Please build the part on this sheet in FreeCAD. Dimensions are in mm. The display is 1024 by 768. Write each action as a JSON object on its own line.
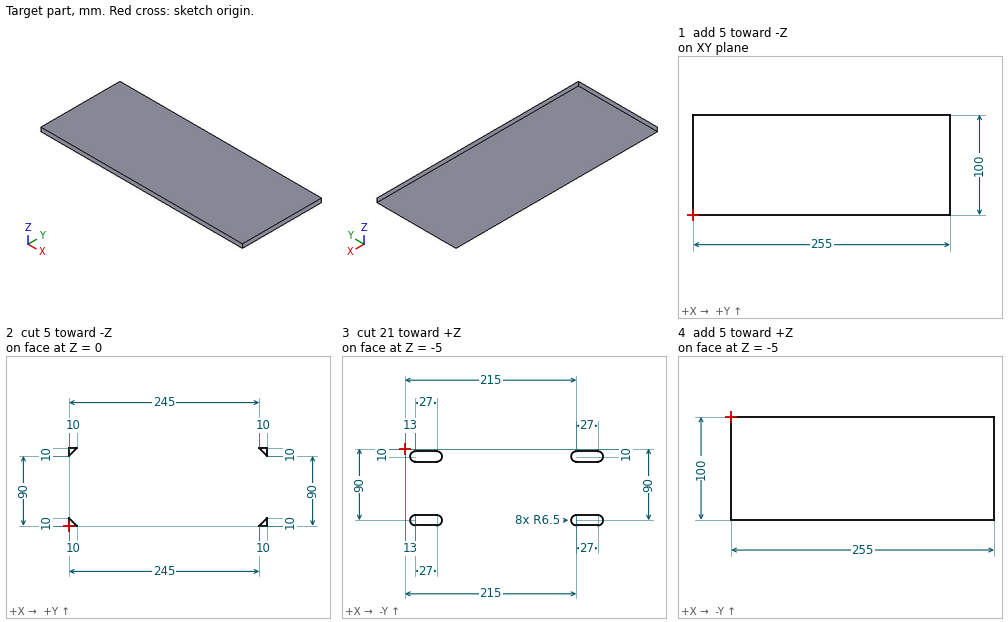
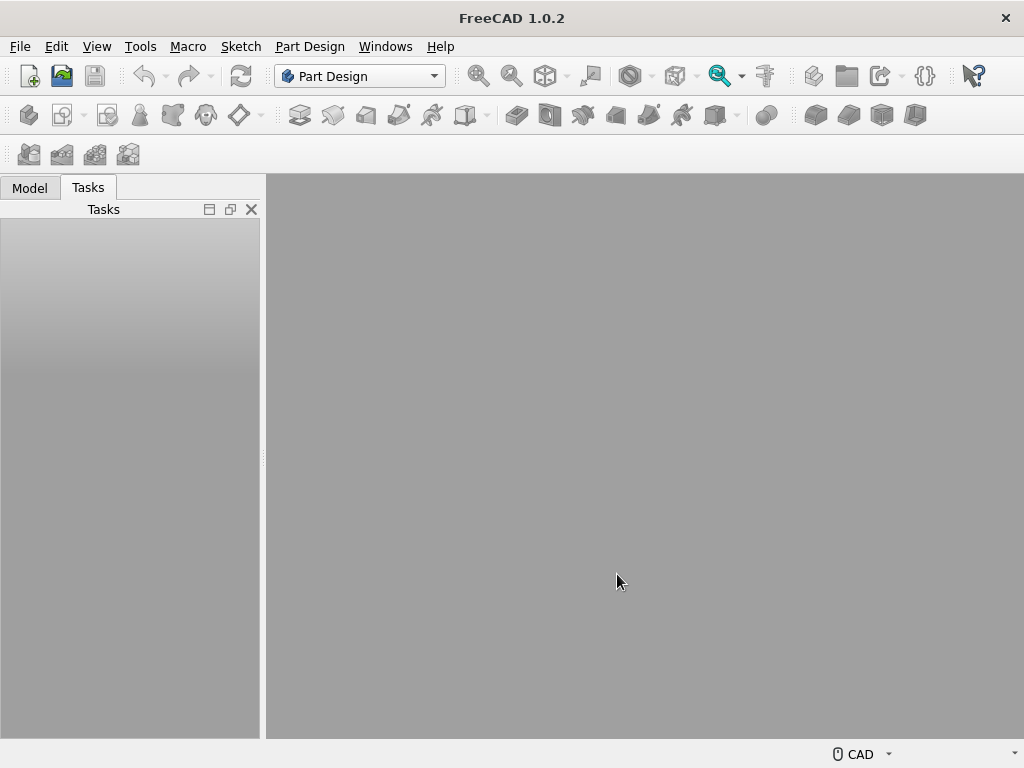
{"action": "key", "text": "ctrl+n"}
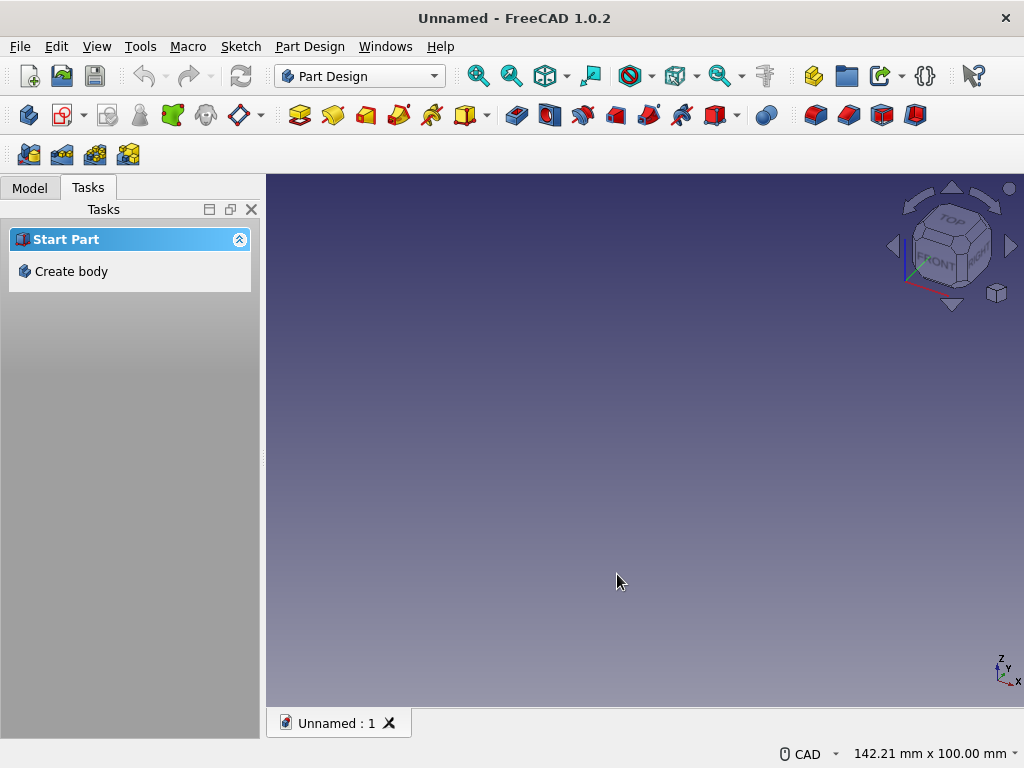
{"action": "left_click", "coordinate": [62, 116]}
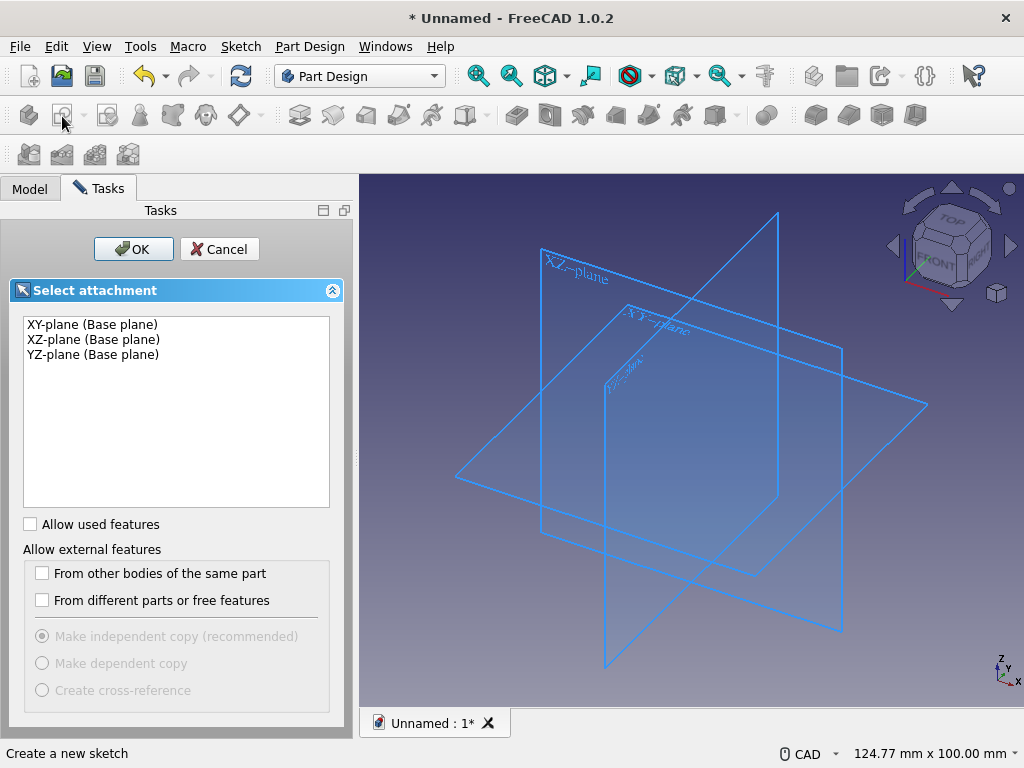
{"action": "left_click", "coordinate": [84, 324]}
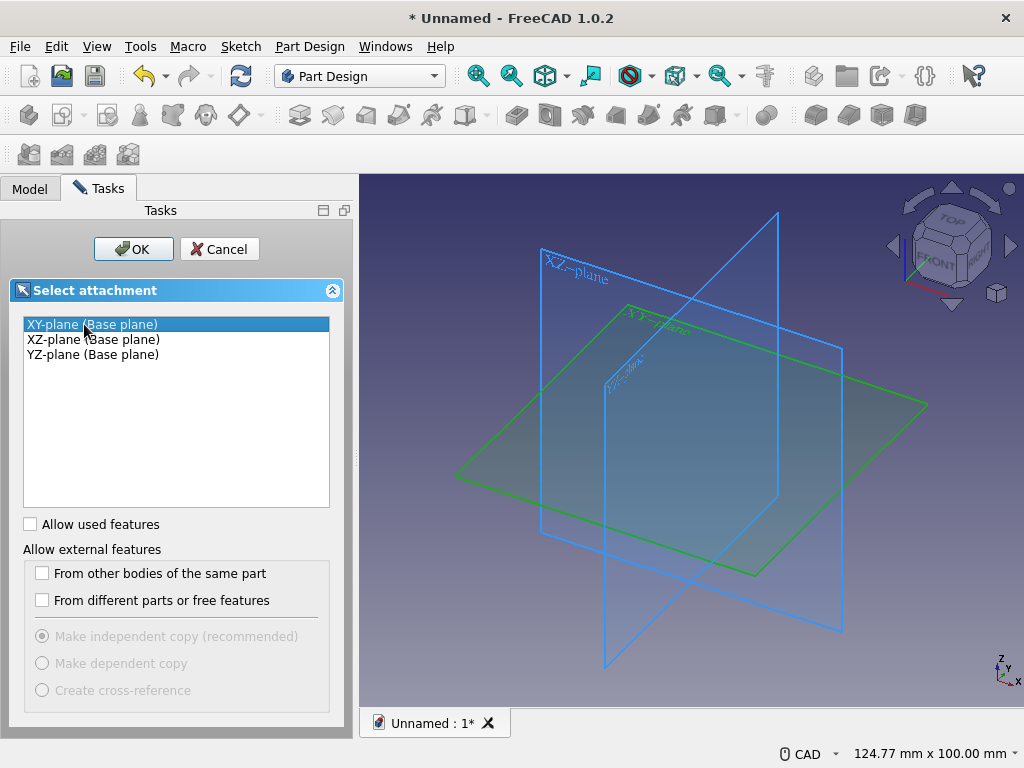
{"action": "left_click", "coordinate": [134, 249]}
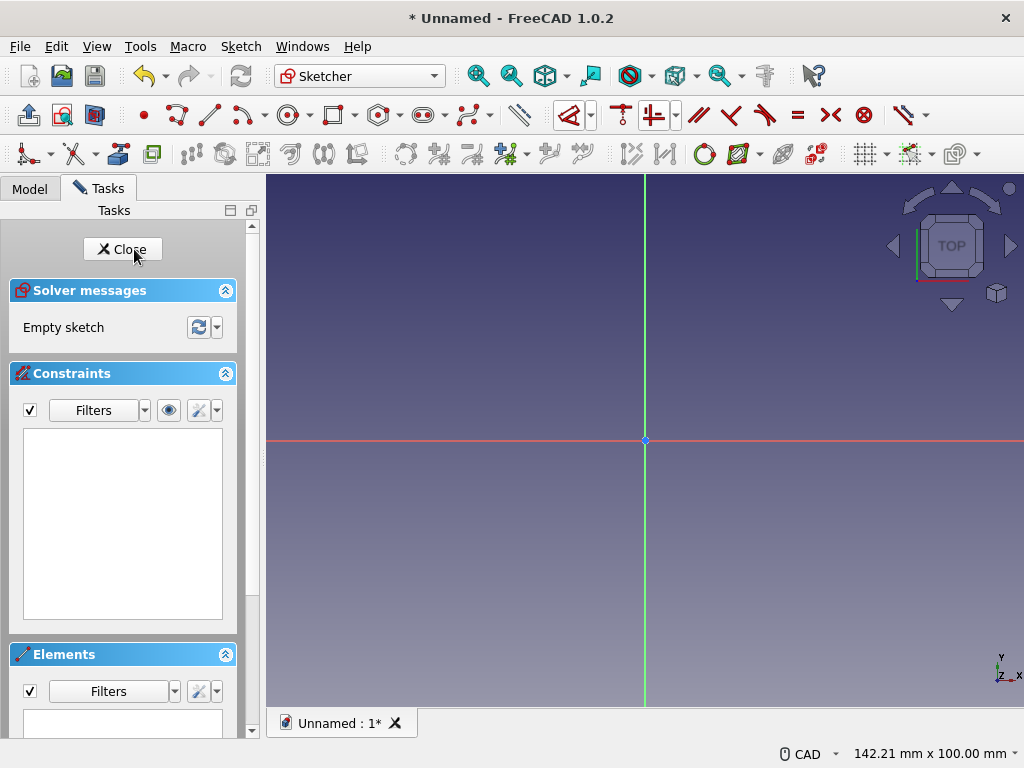
{"action": "scroll", "coordinate": [294, 555], "scroll_direction": "down", "scroll_amount": 6}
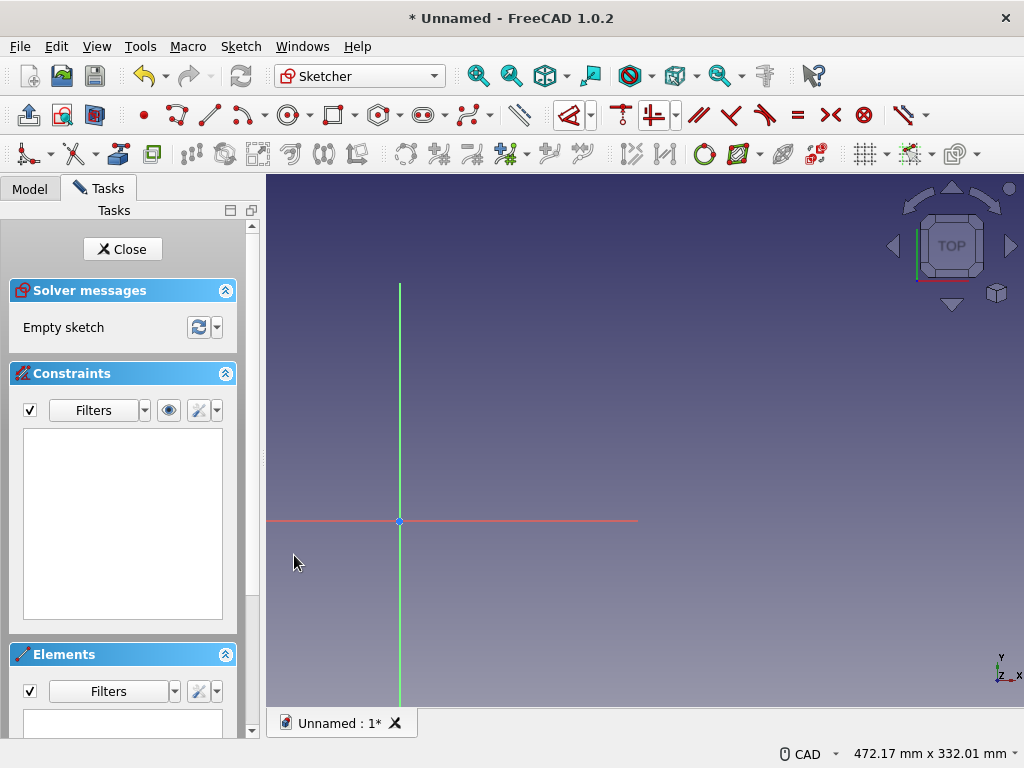
{"action": "left_click", "coordinate": [332, 116]}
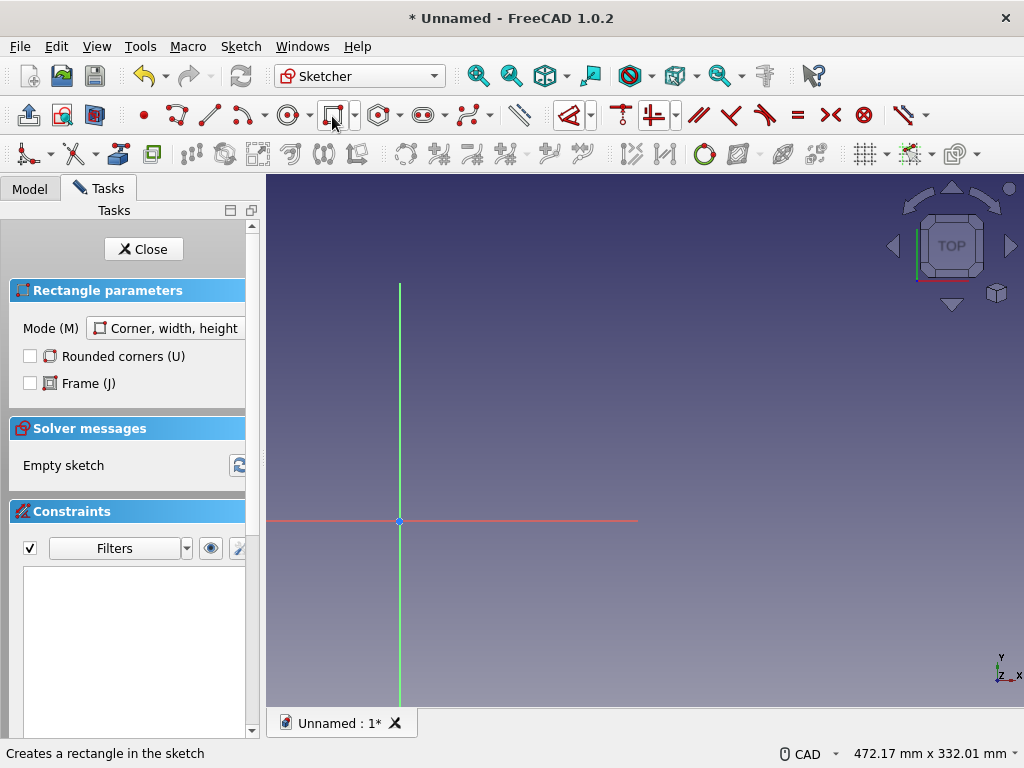
{"action": "left_click", "coordinate": [400, 521]}
{"action": "left_click", "coordinate": [809, 360]}
{"action": "key", "text": "Escape"}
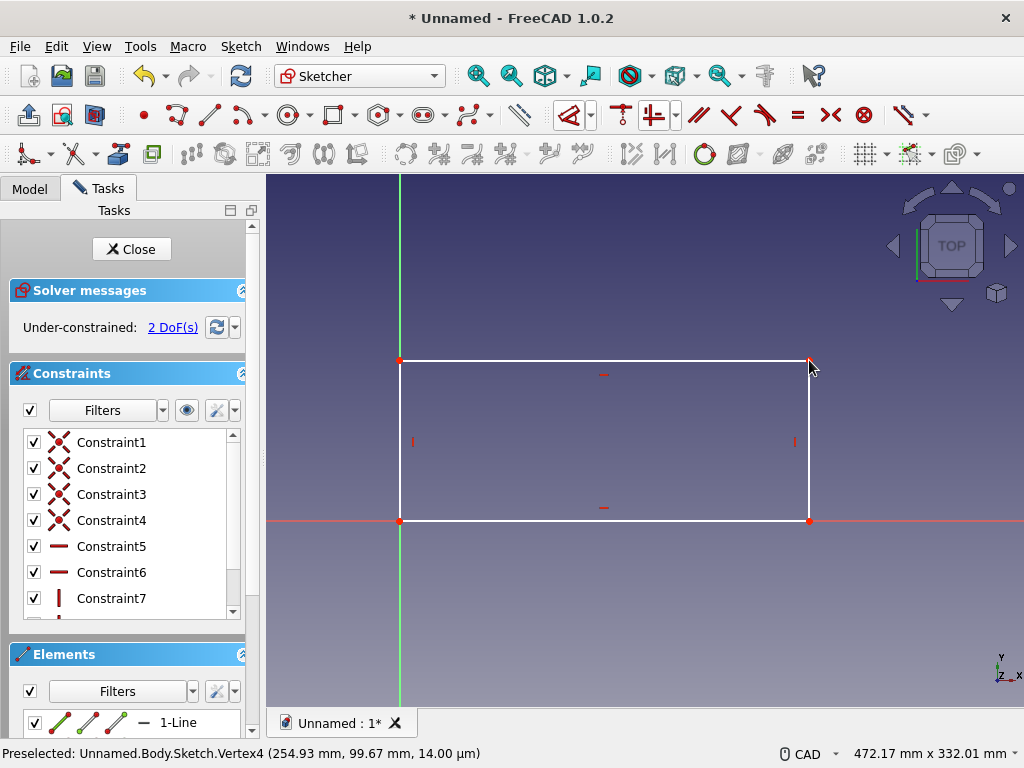
{"action": "key", "text": "d"}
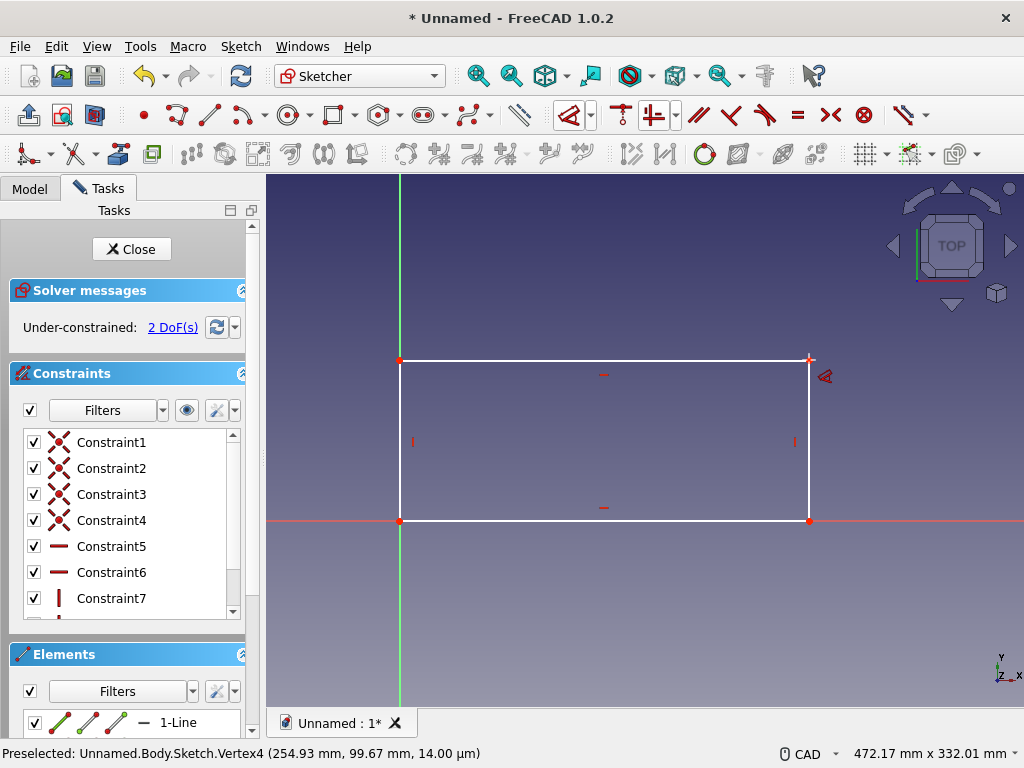
{"action": "left_click", "coordinate": [523, 521]}
{"action": "left_click", "coordinate": [604, 555]}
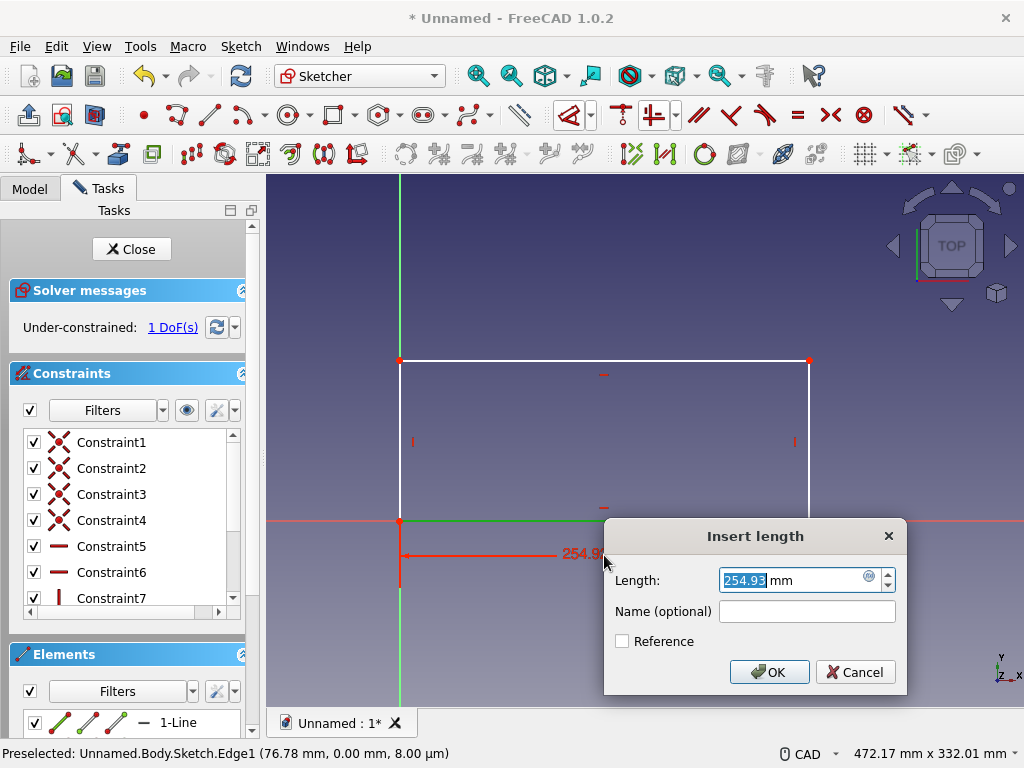
{"action": "type", "text": "255"}
{"action": "key", "text": "Return"}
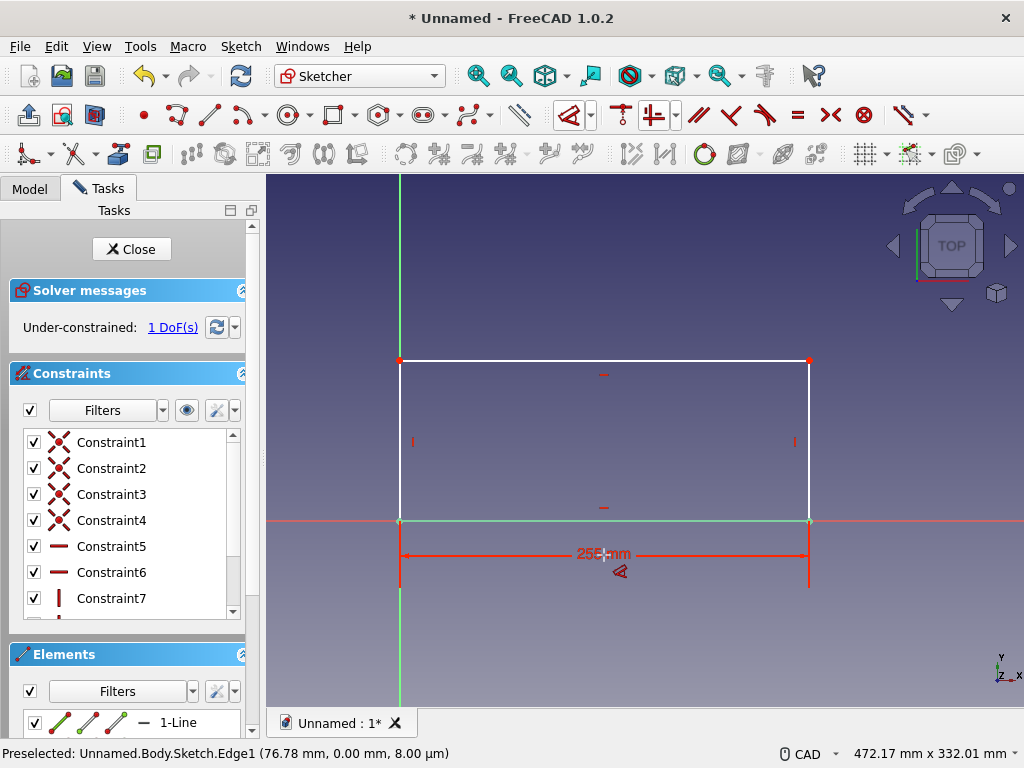
{"action": "left_click", "coordinate": [809, 473]}
{"action": "left_click", "coordinate": [843, 441]}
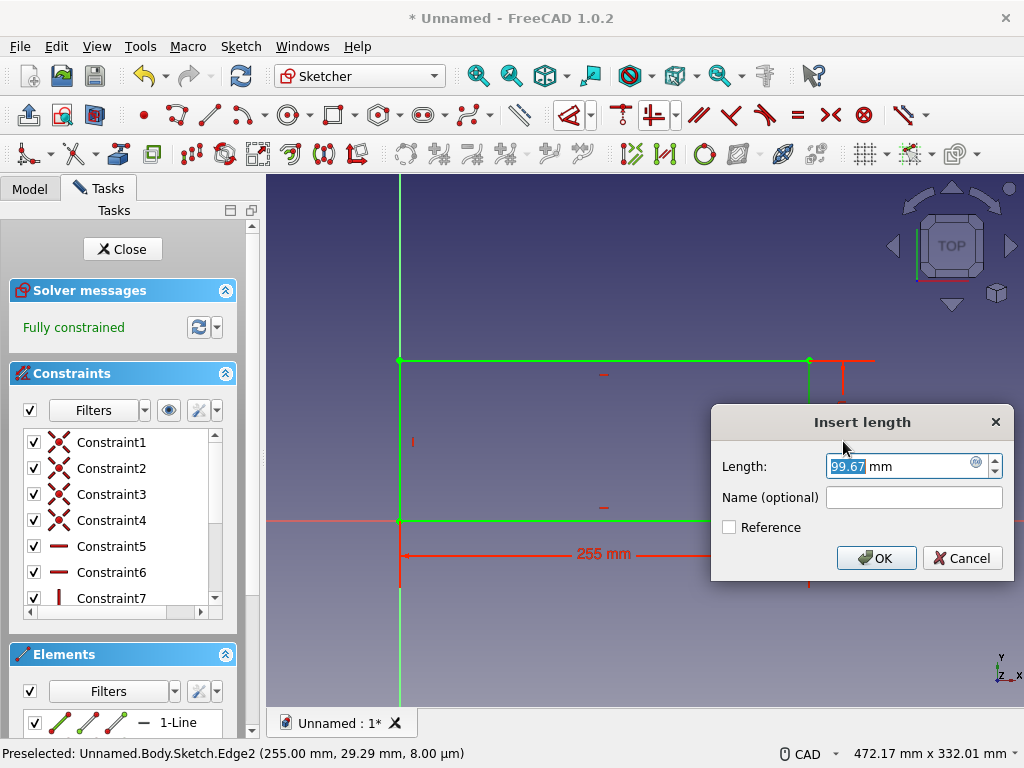
{"action": "type", "text": "100"}
{"action": "key", "text": "Return"}
{"action": "key", "text": "Escape"}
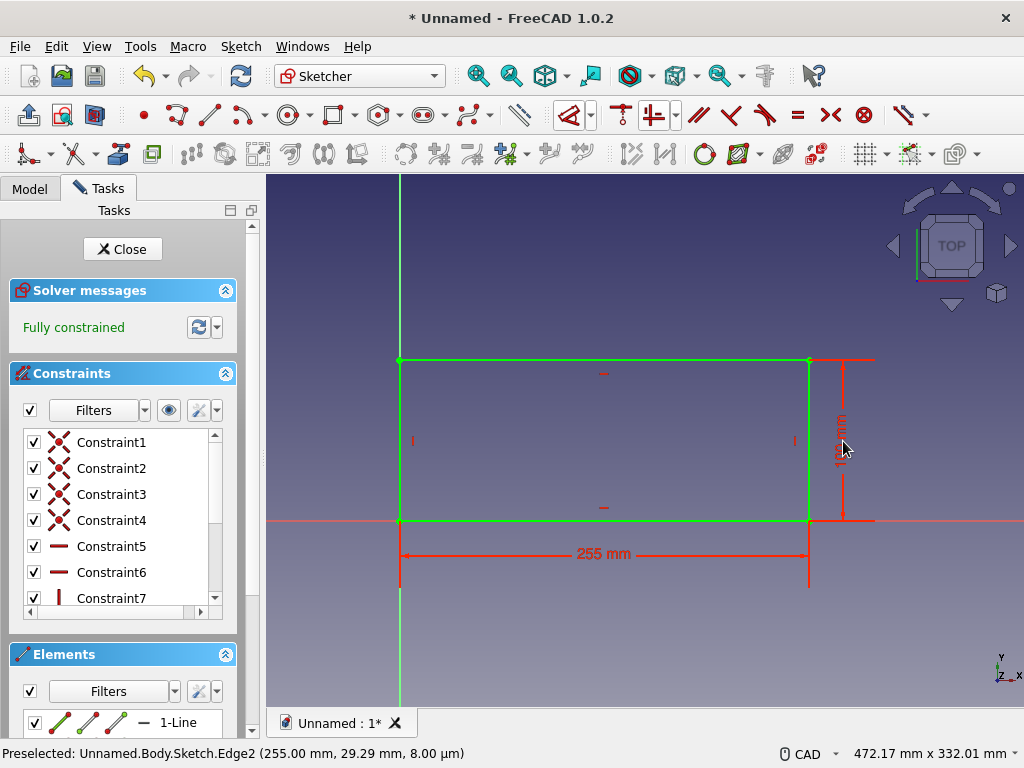
{"action": "left_click", "coordinate": [123, 249]}